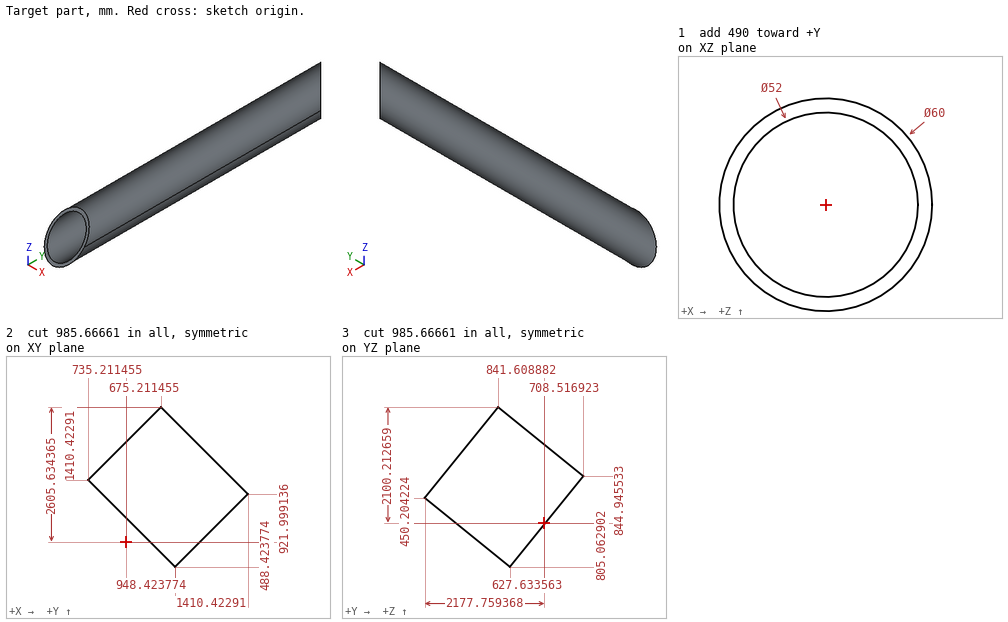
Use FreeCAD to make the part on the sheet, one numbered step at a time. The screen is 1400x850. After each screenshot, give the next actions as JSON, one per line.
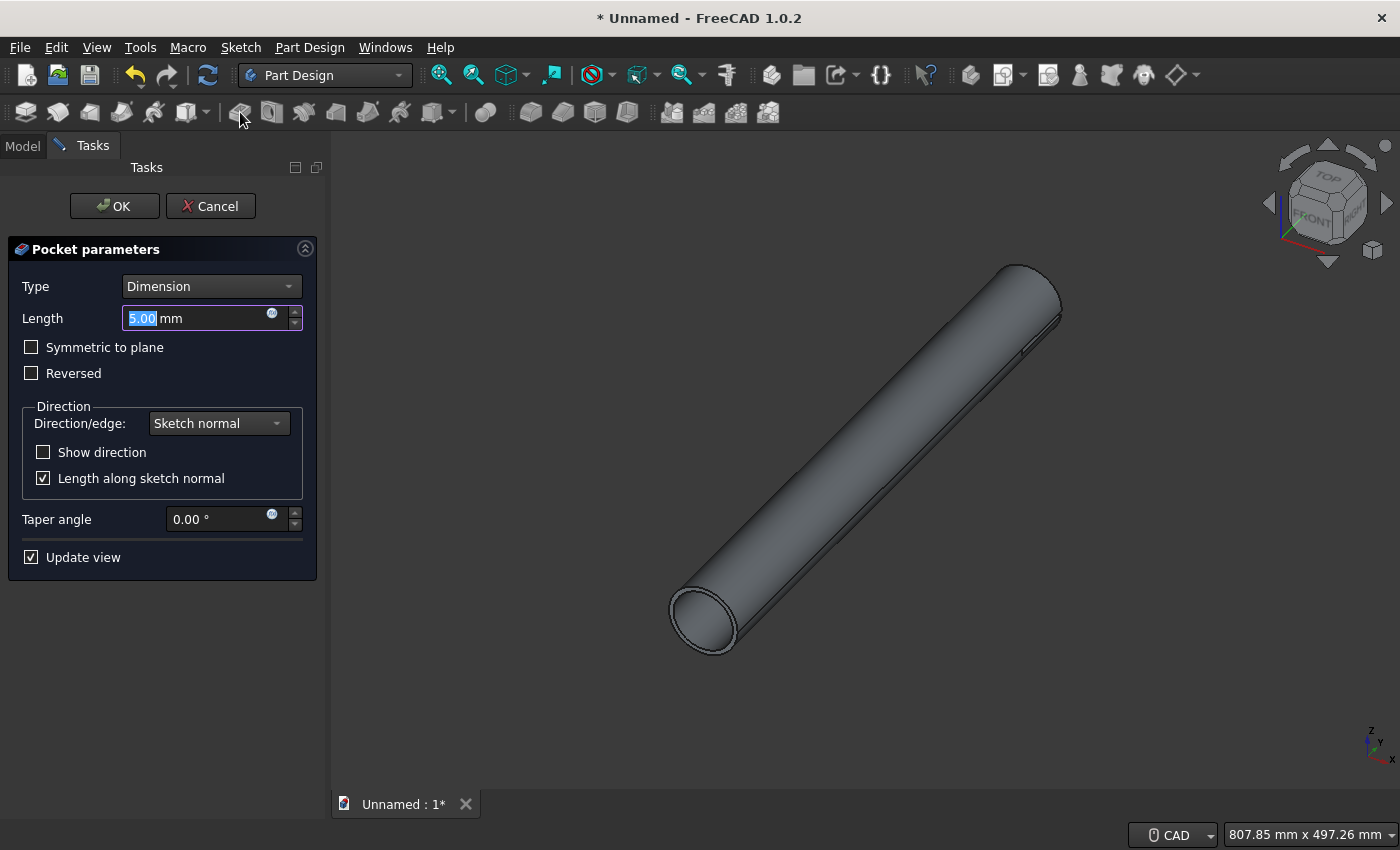
{"action": "type", "text": "985.66661"}
{"action": "key", "text": "Tab"}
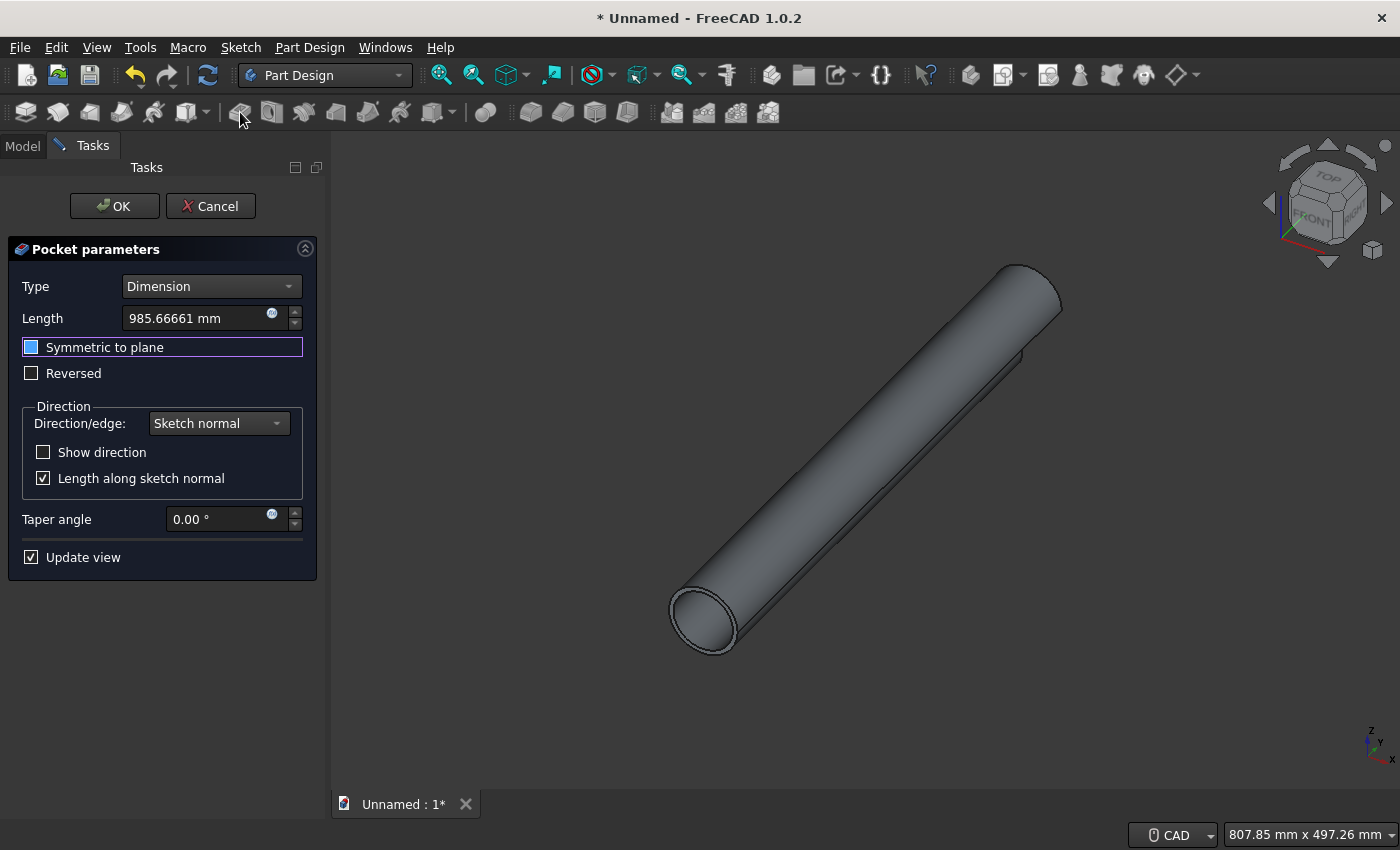
{"action": "left_click", "coordinate": [30, 347]}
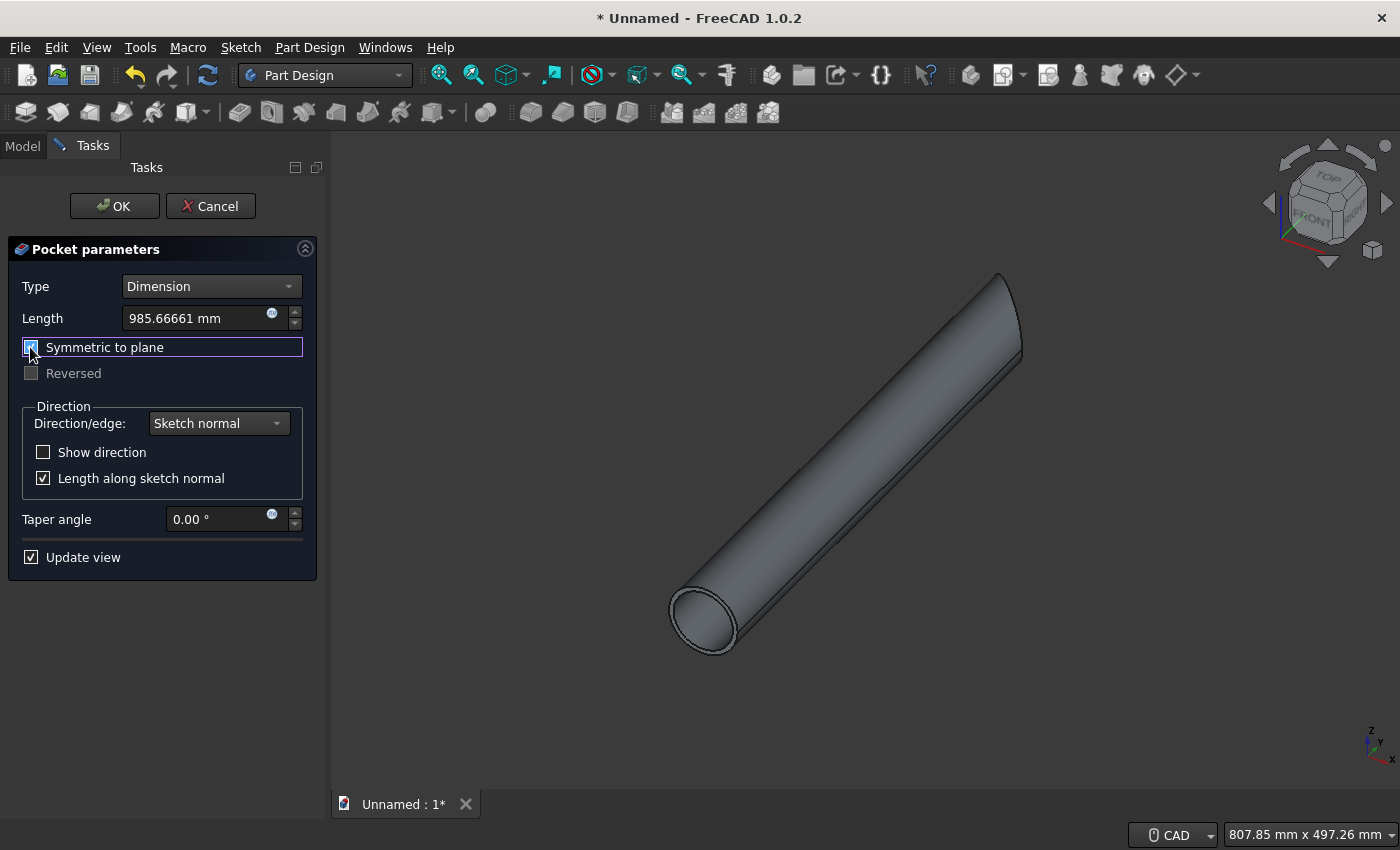
{"action": "left_click", "coordinate": [115, 206]}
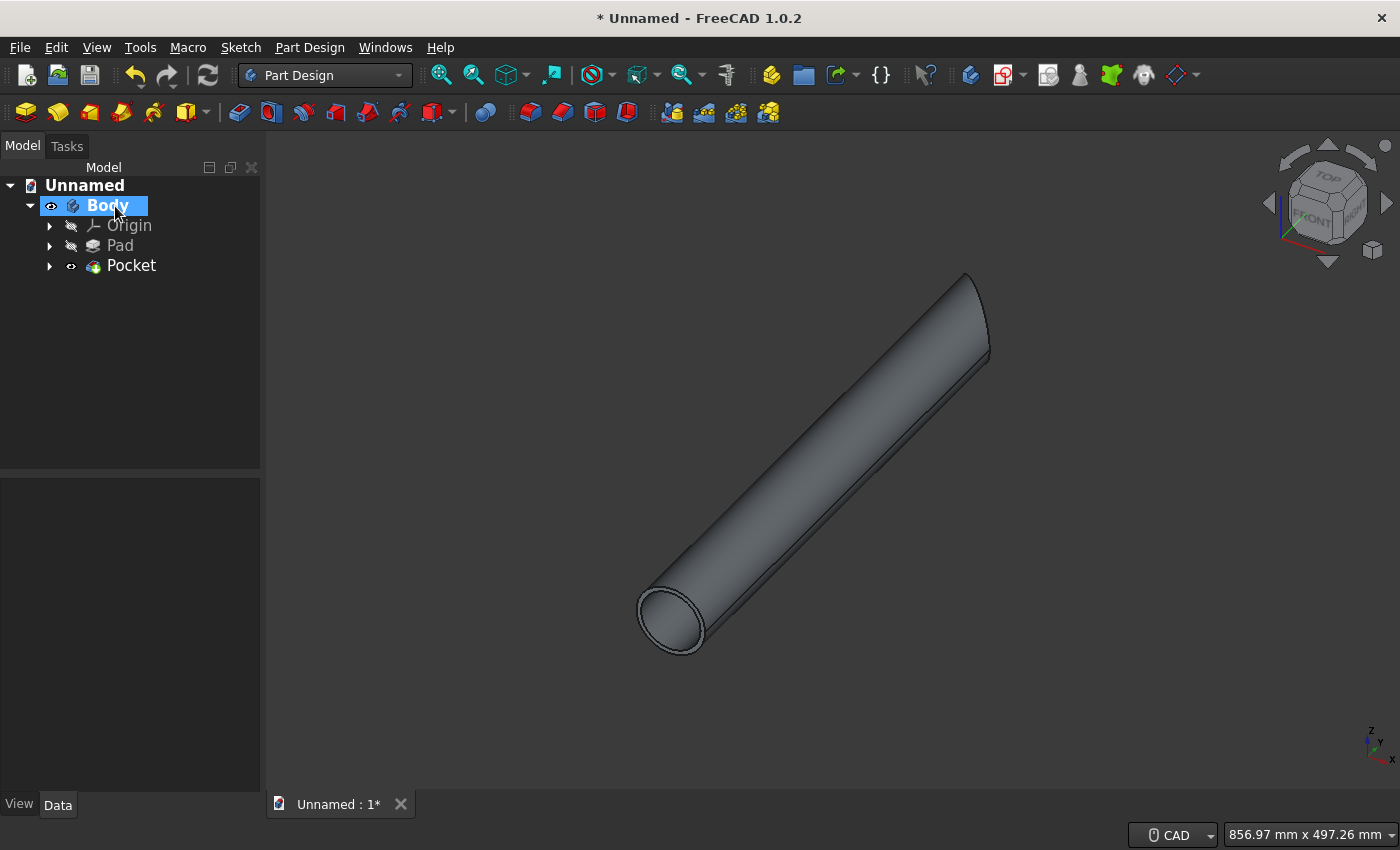
{"action": "left_click", "coordinate": [1004, 76]}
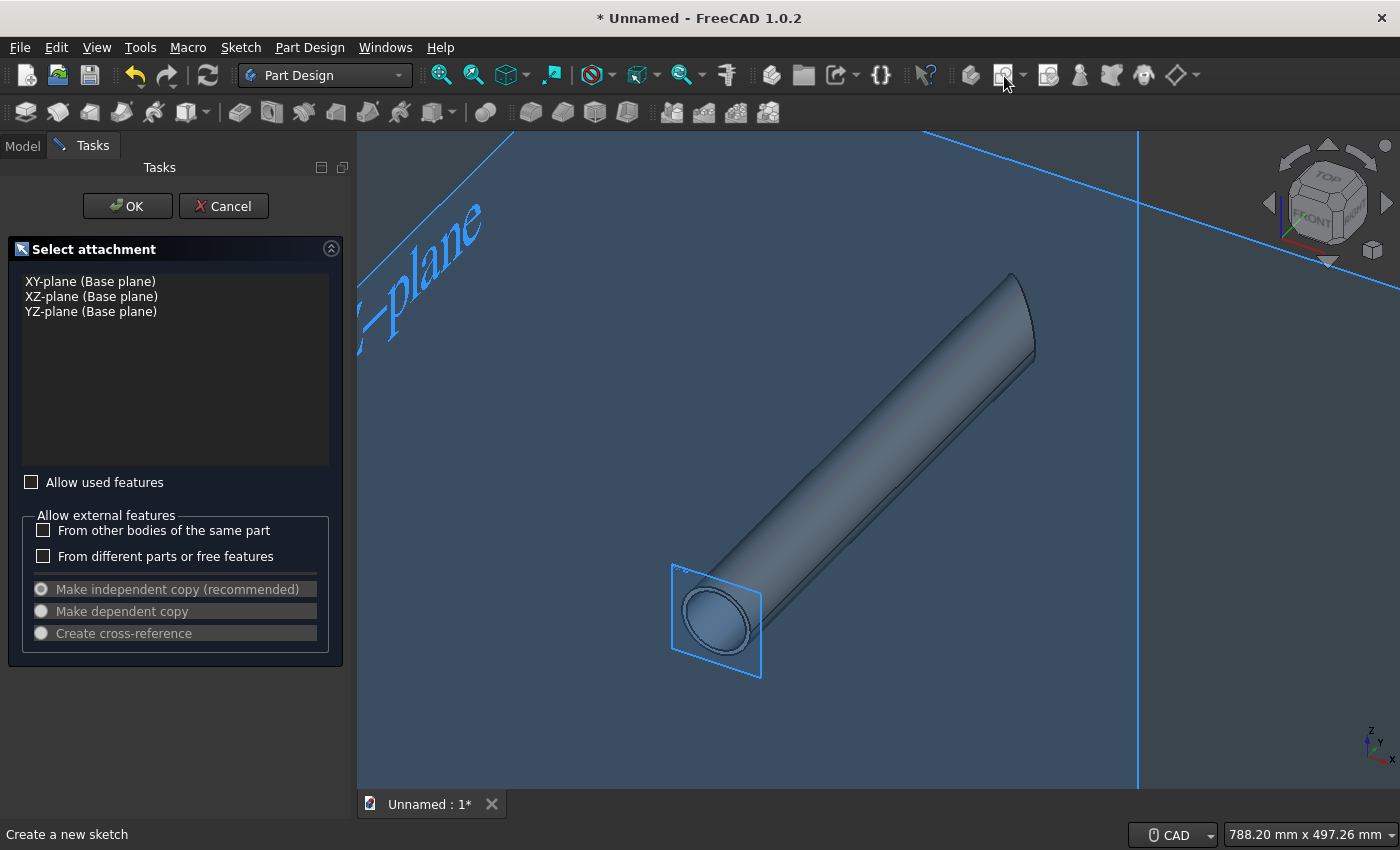
{"action": "left_click", "coordinate": [82, 312]}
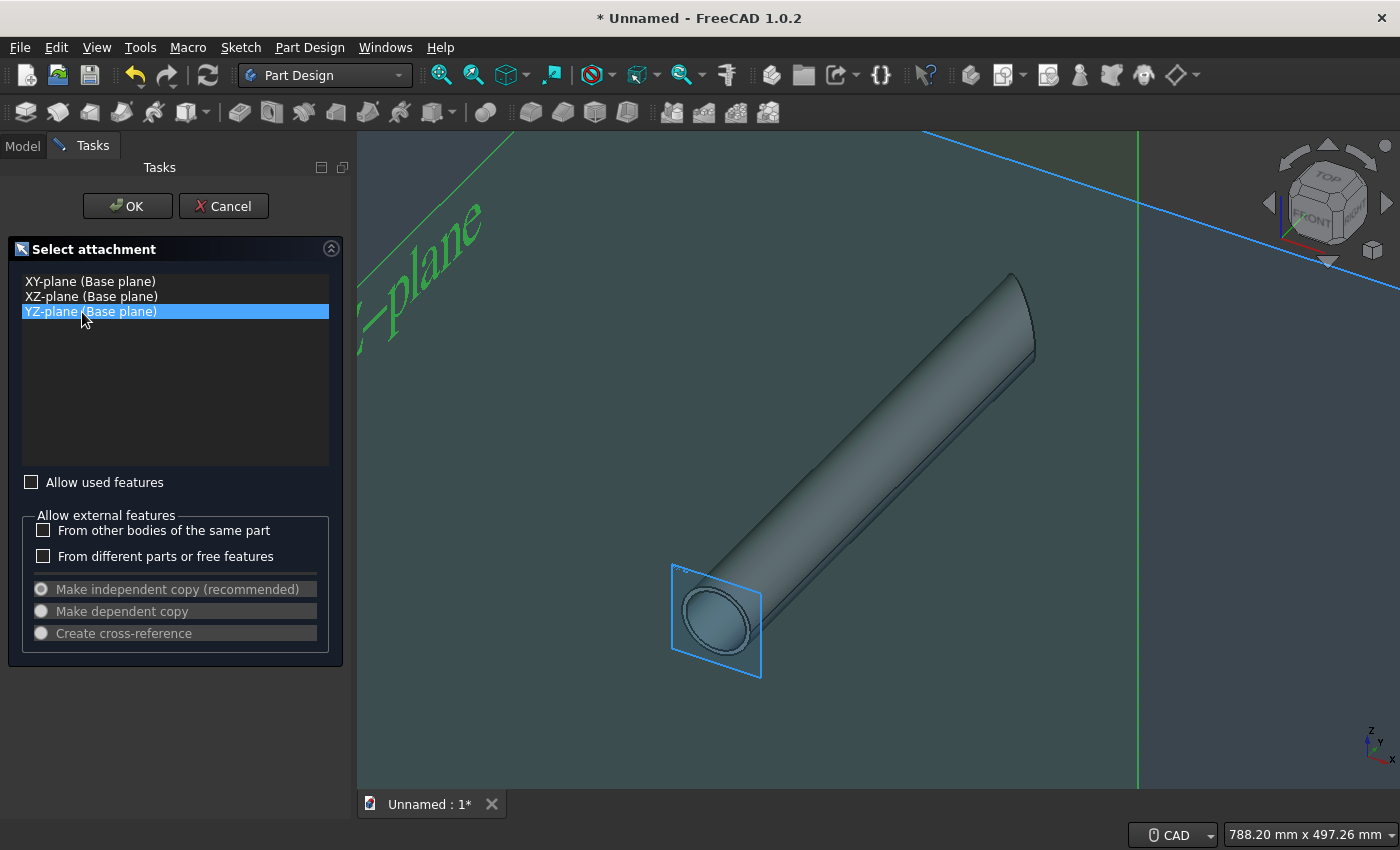
{"action": "left_click", "coordinate": [128, 206]}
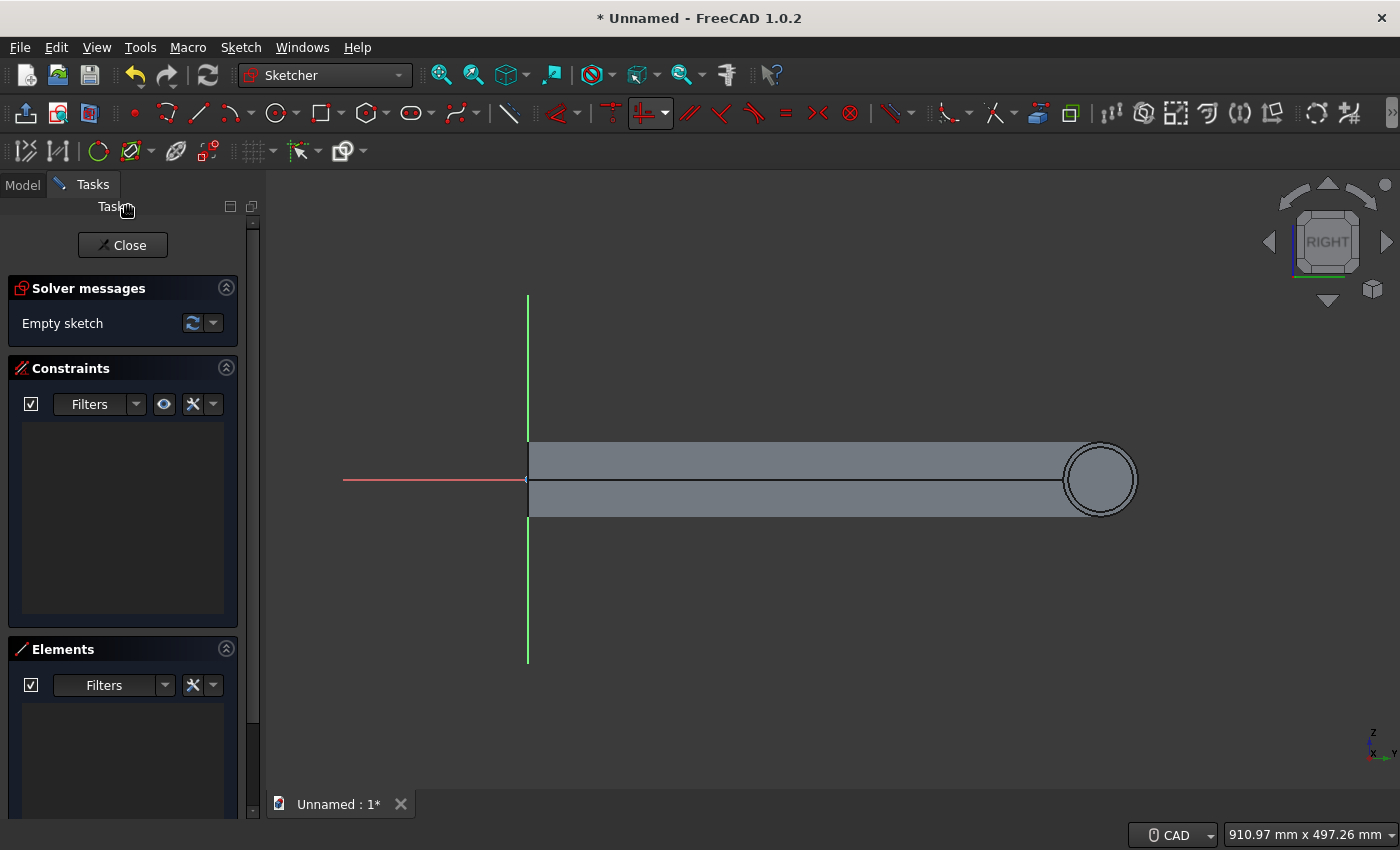
{"action": "key", "text": "q s"}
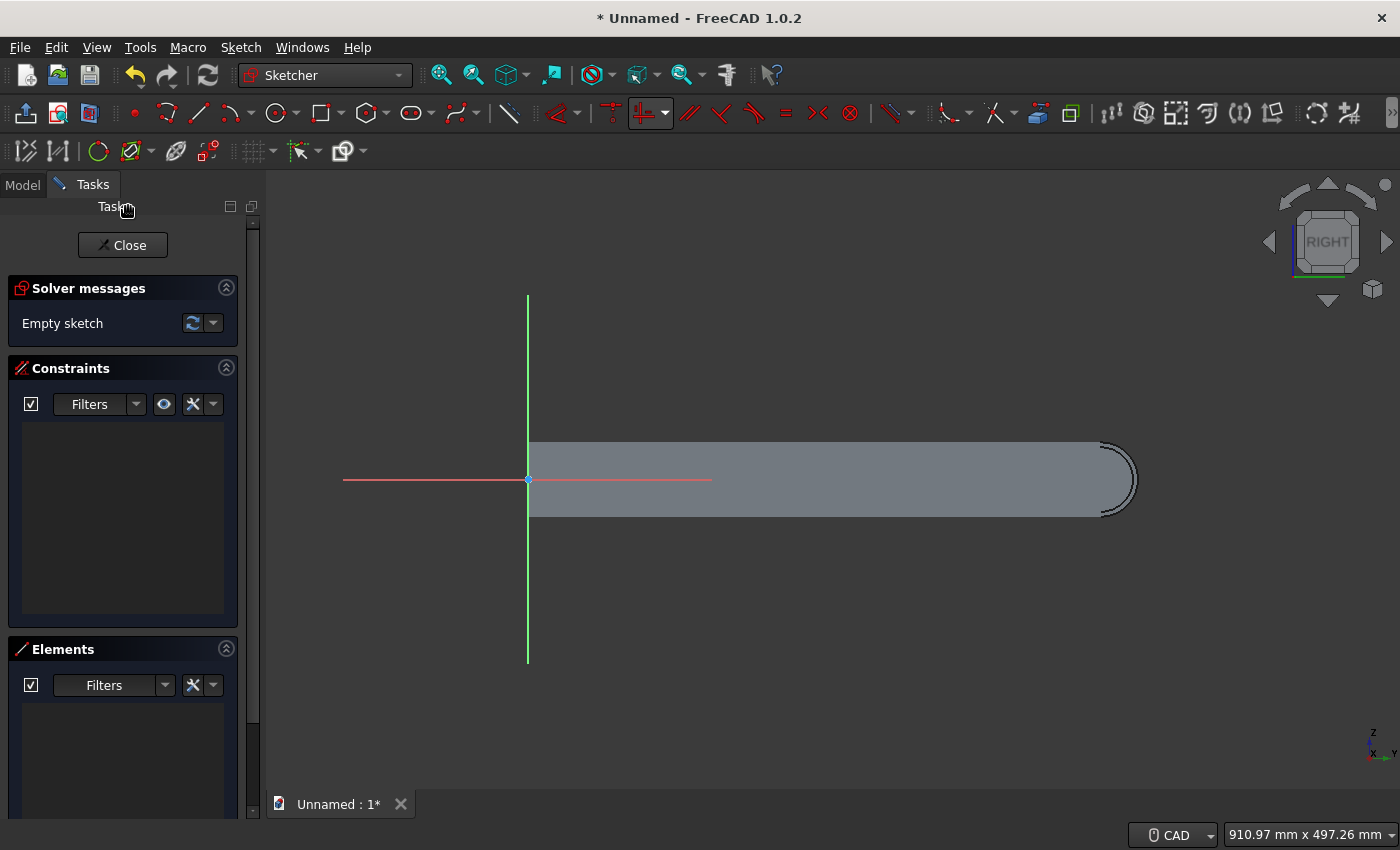
{"action": "scroll", "coordinate": [908, 580], "scroll_direction": "down", "scroll_amount": 11}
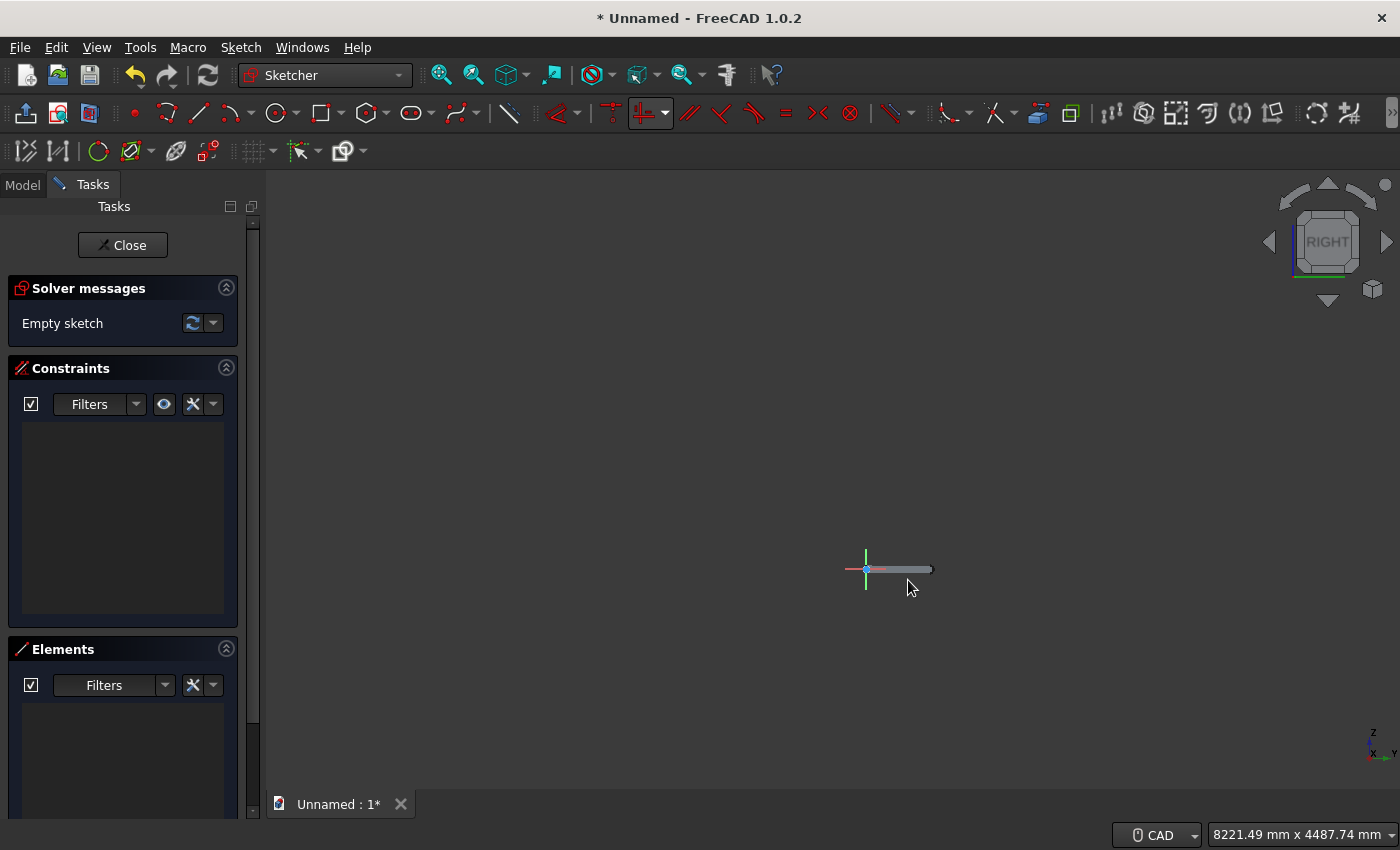
{"action": "key", "text": "g m"}